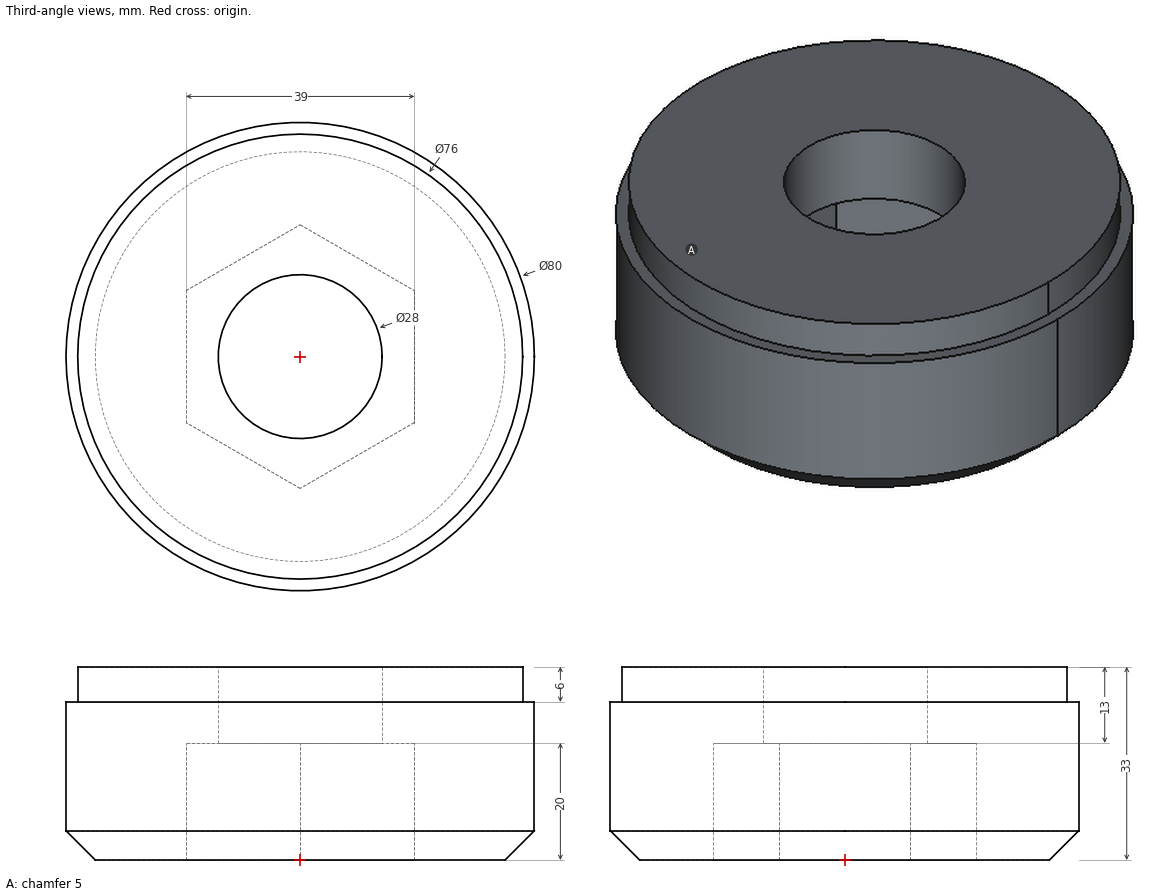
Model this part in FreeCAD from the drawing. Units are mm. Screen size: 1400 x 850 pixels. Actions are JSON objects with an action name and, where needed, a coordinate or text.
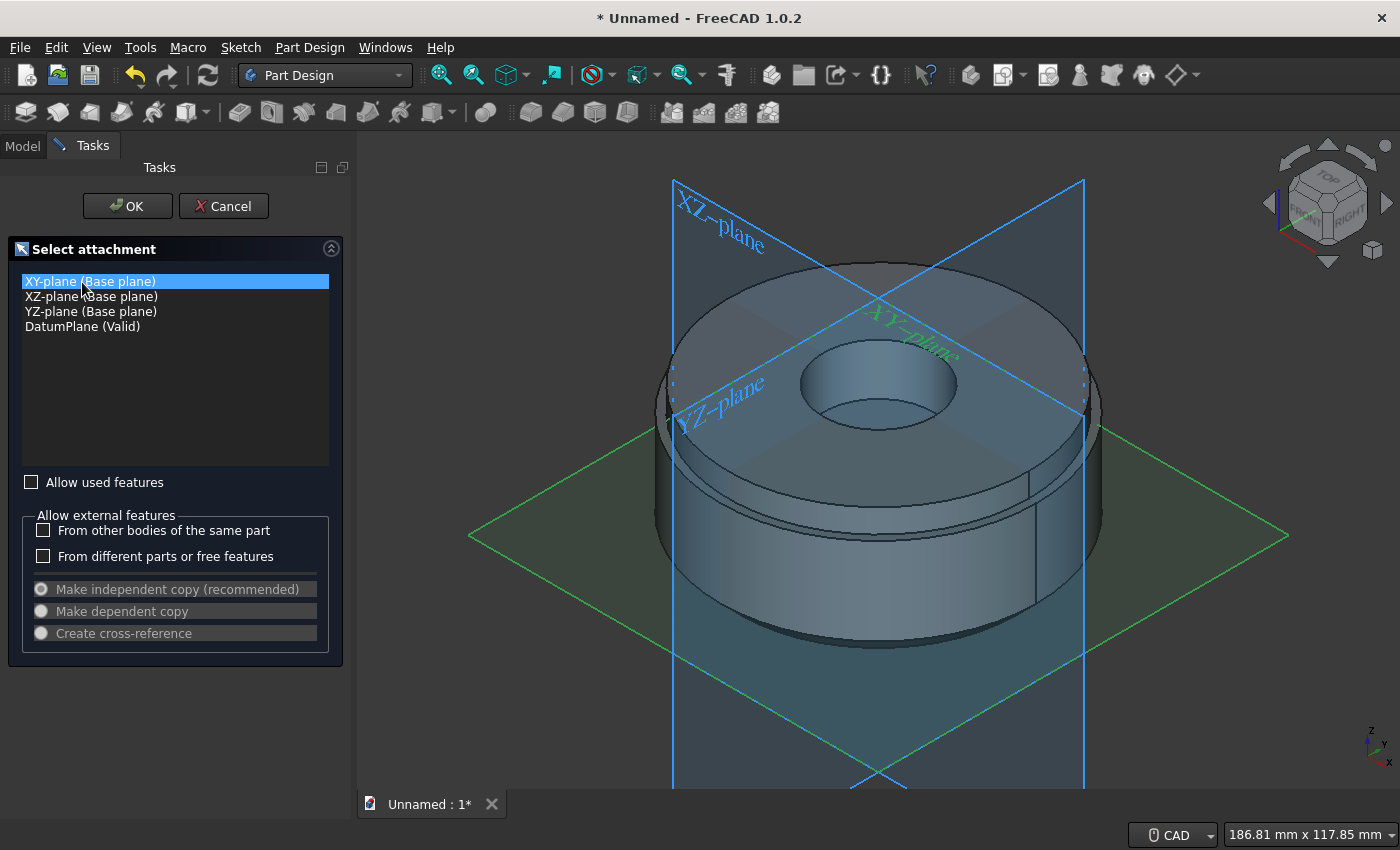
{"action": "left_click", "coordinate": [128, 206]}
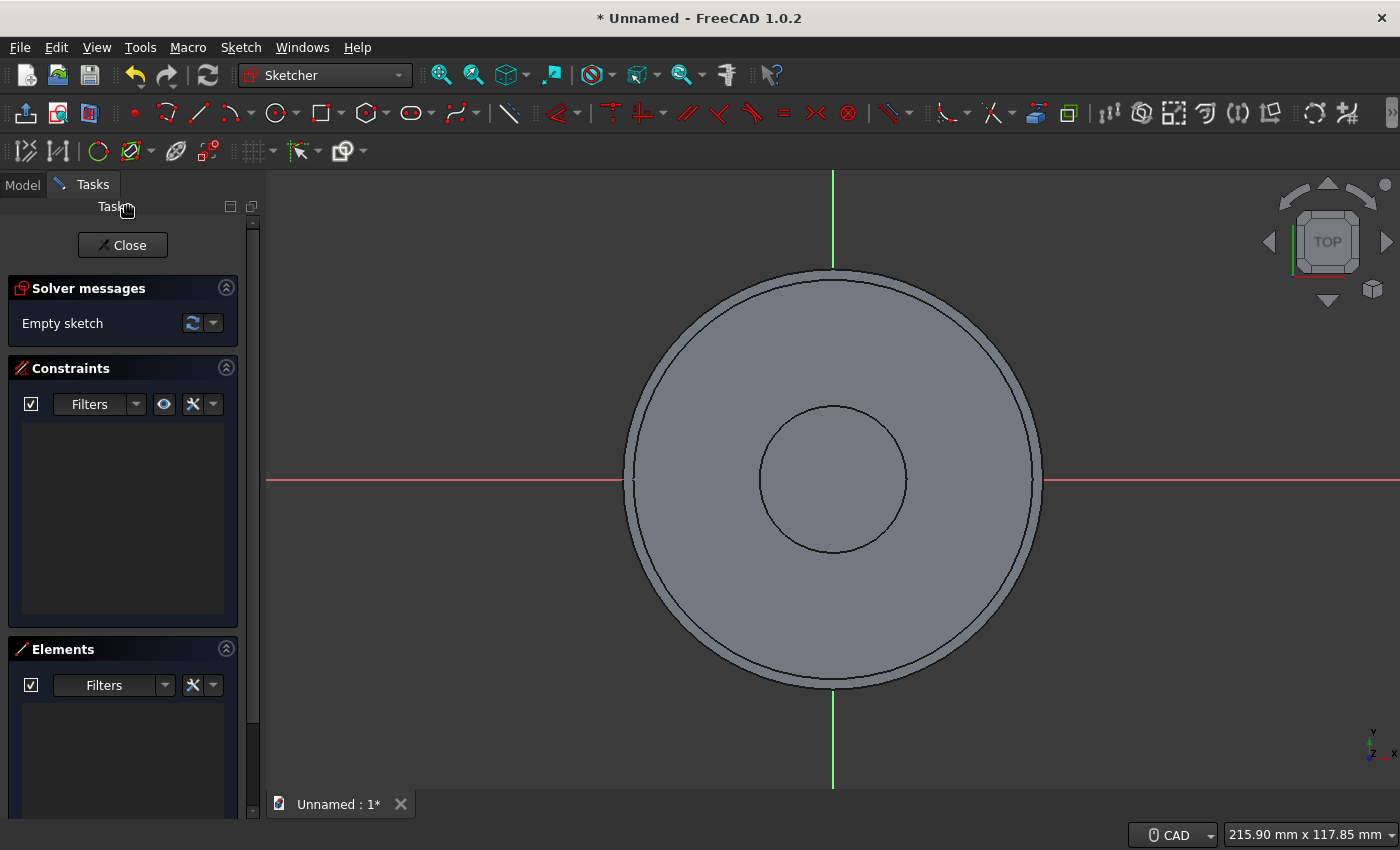
{"action": "left_click", "coordinate": [90, 114]}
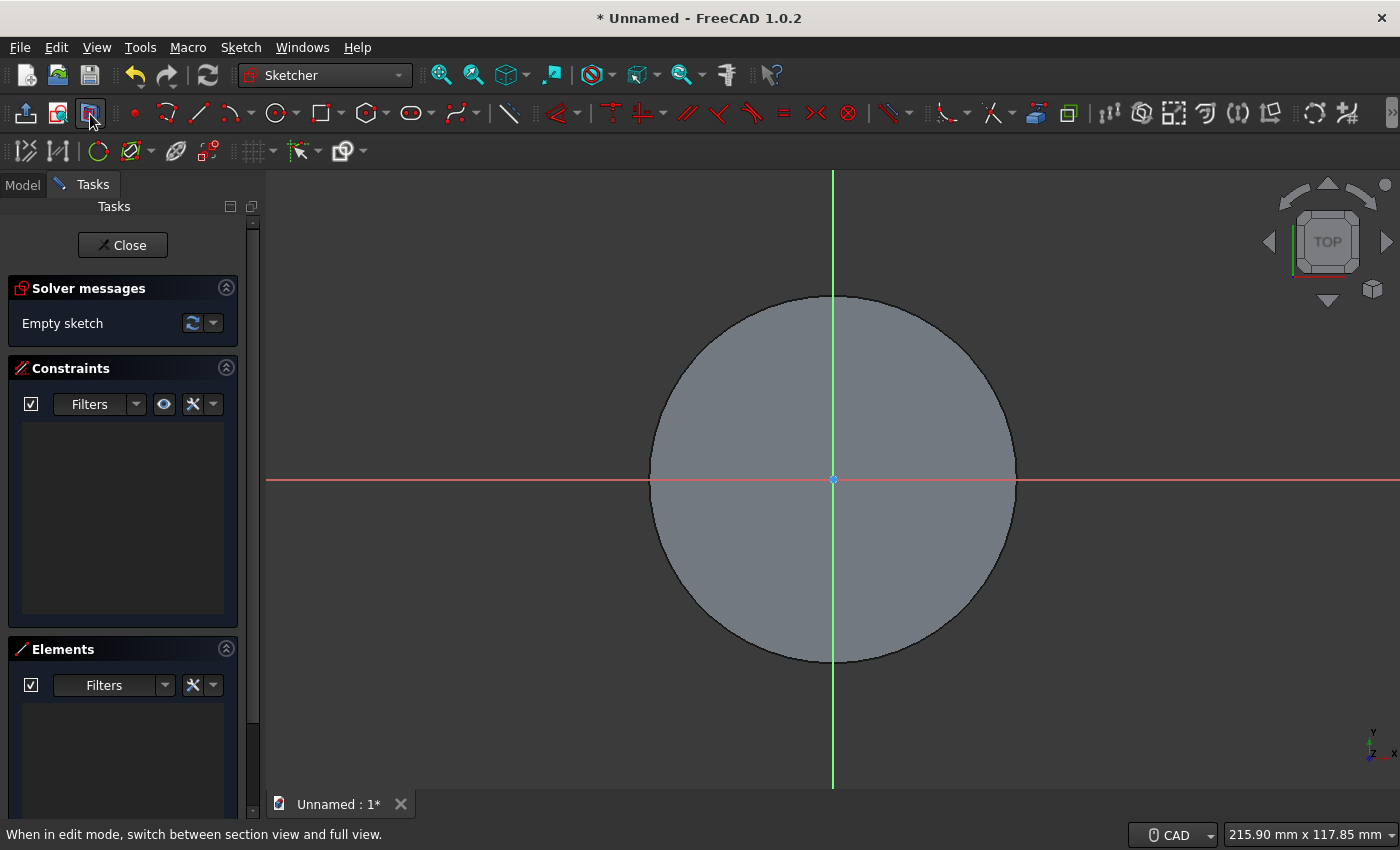
{"action": "scroll", "coordinate": [916, 480], "scroll_direction": "up", "scroll_amount": 3}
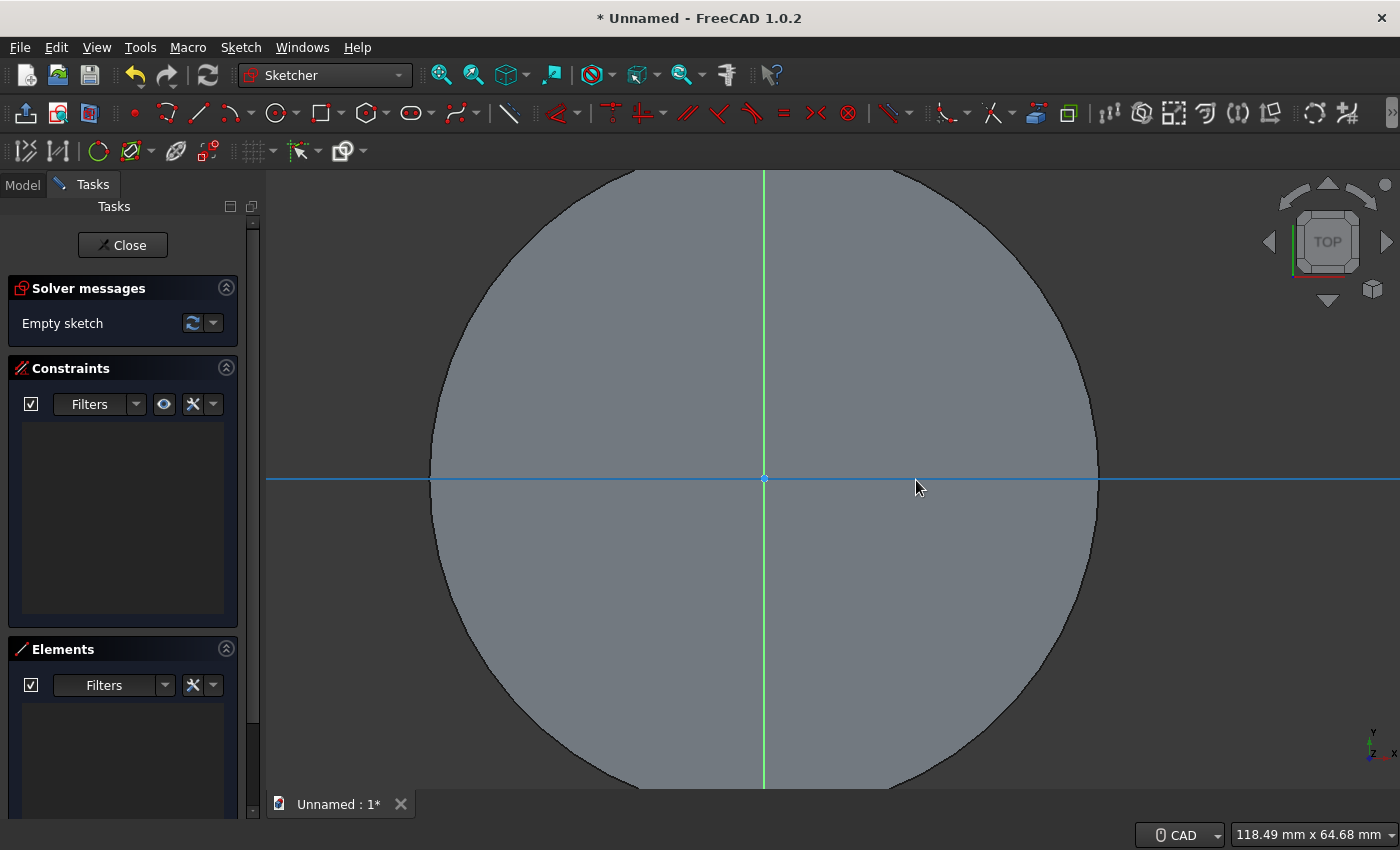
{"action": "left_click", "coordinate": [366, 114]}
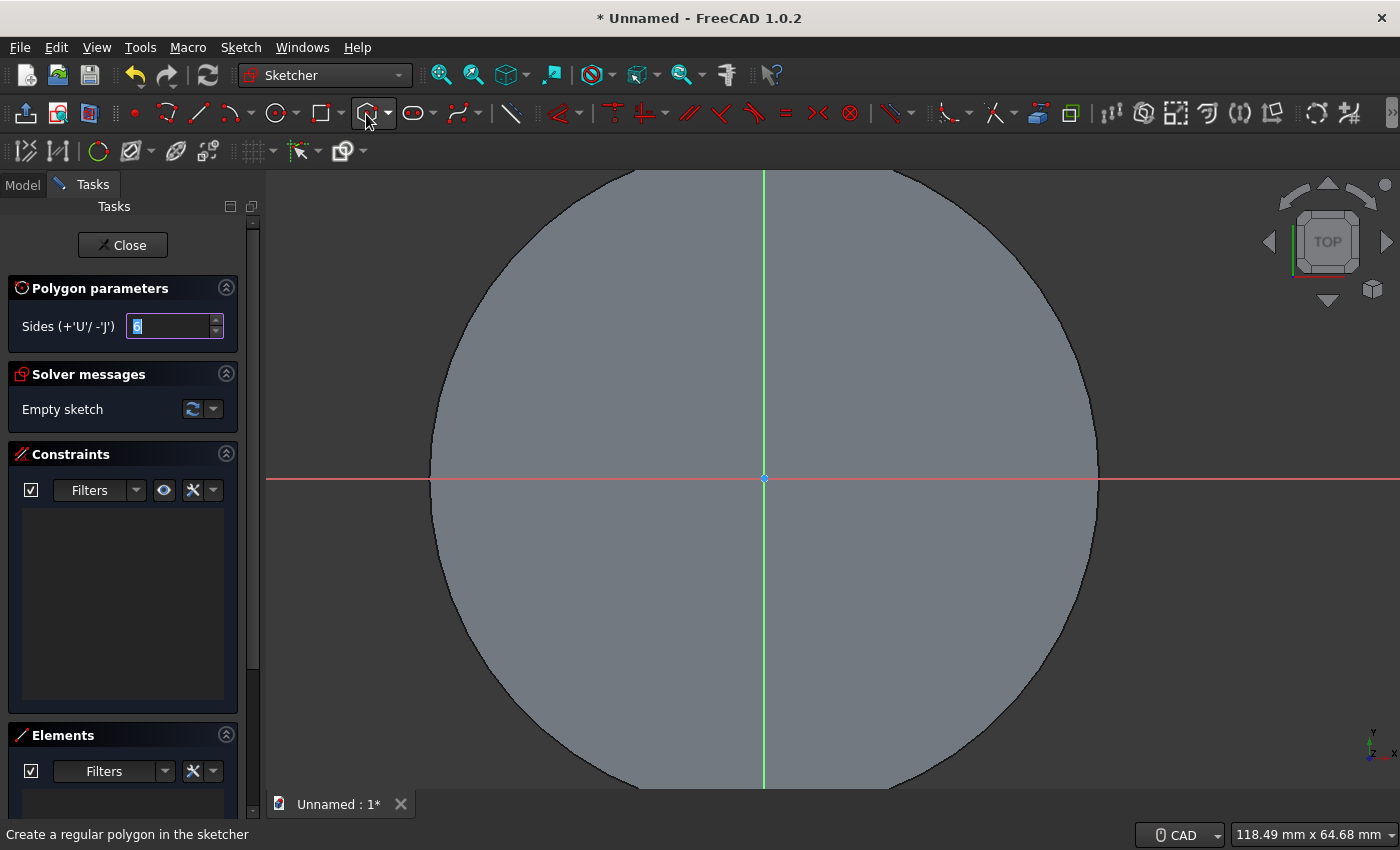
{"action": "left_click", "coordinate": [764, 479]}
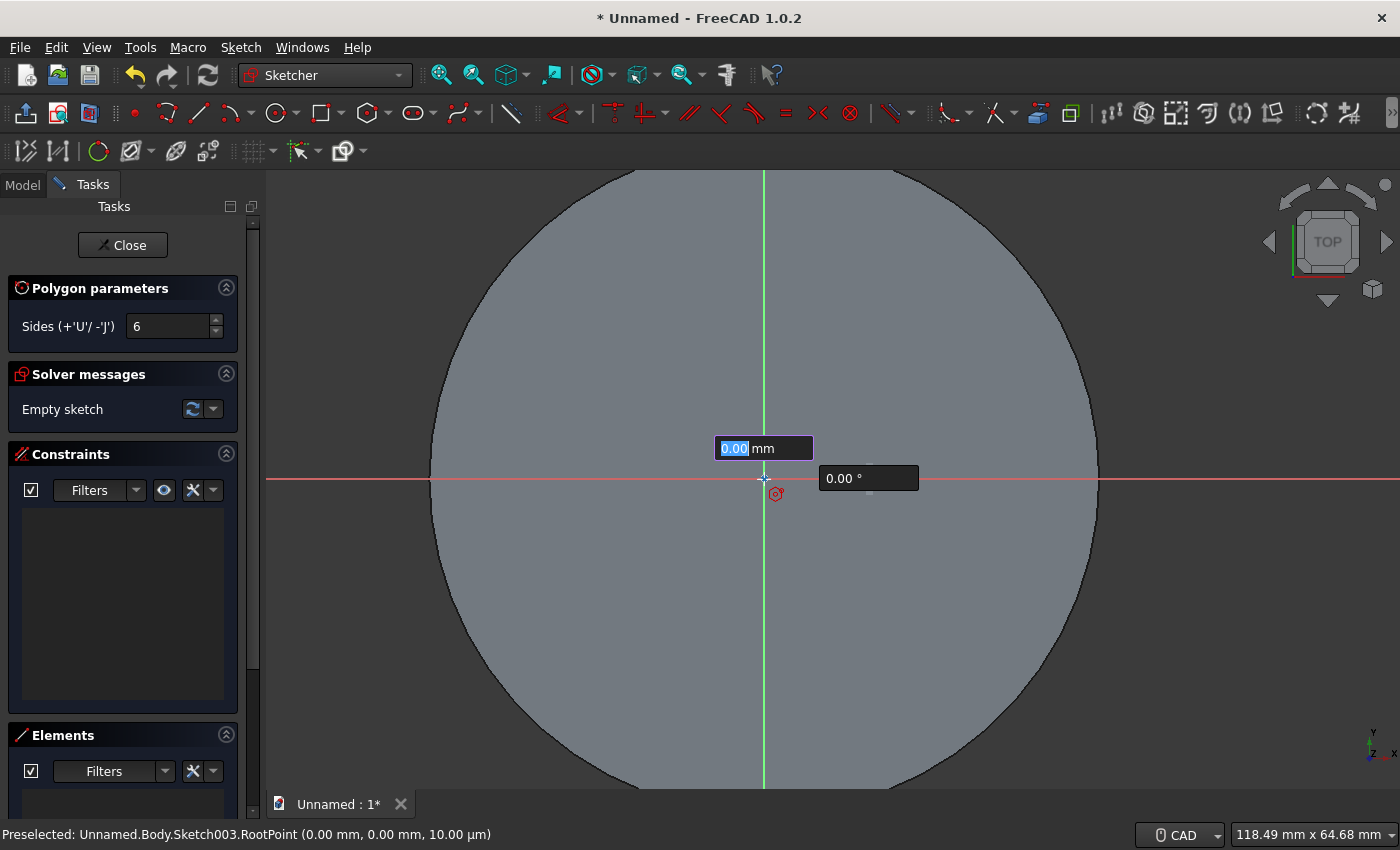
{"action": "left_click", "coordinate": [764, 694]}
{"action": "right_click", "coordinate": [764, 694]}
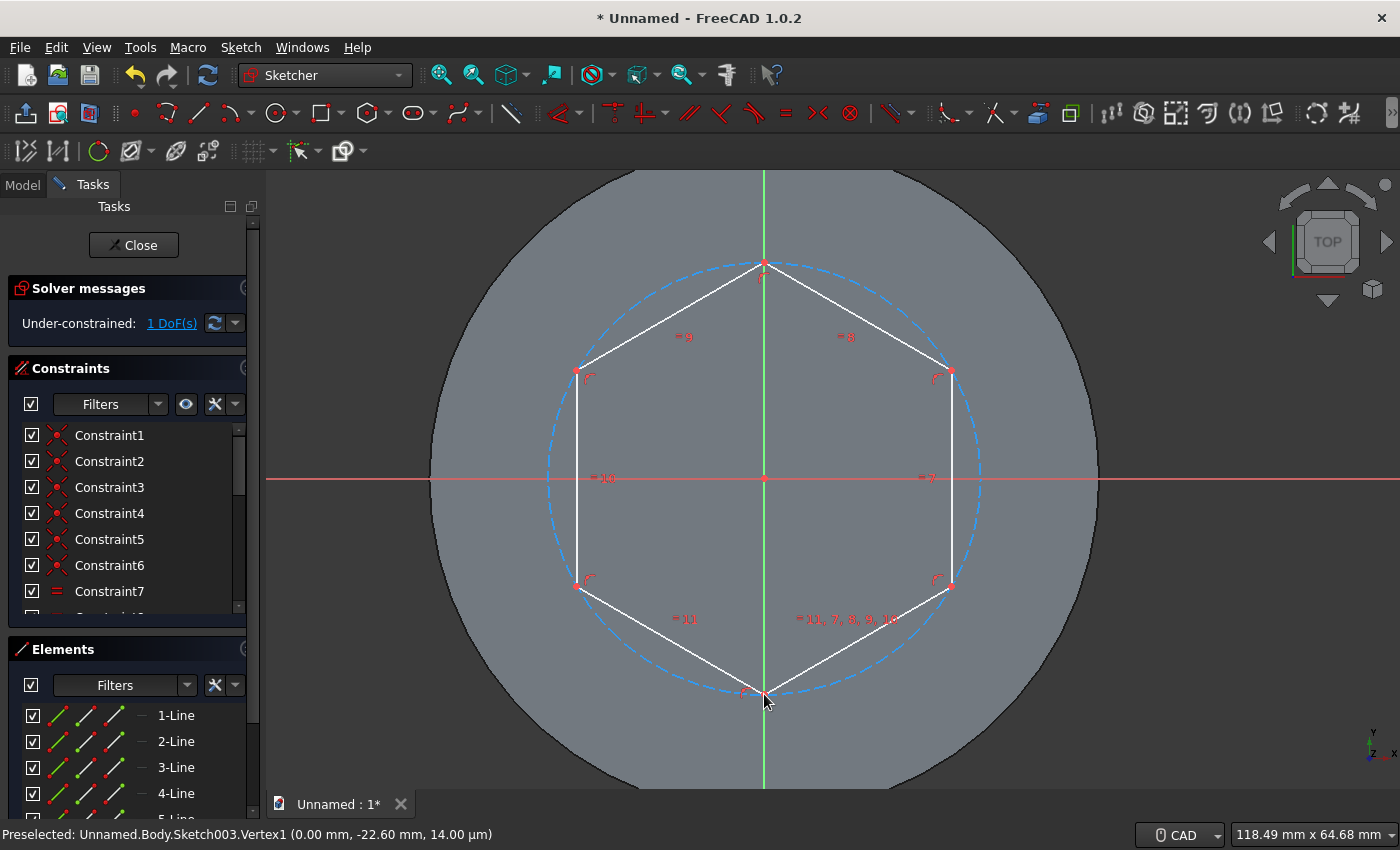
{"action": "left_click", "coordinate": [558, 114]}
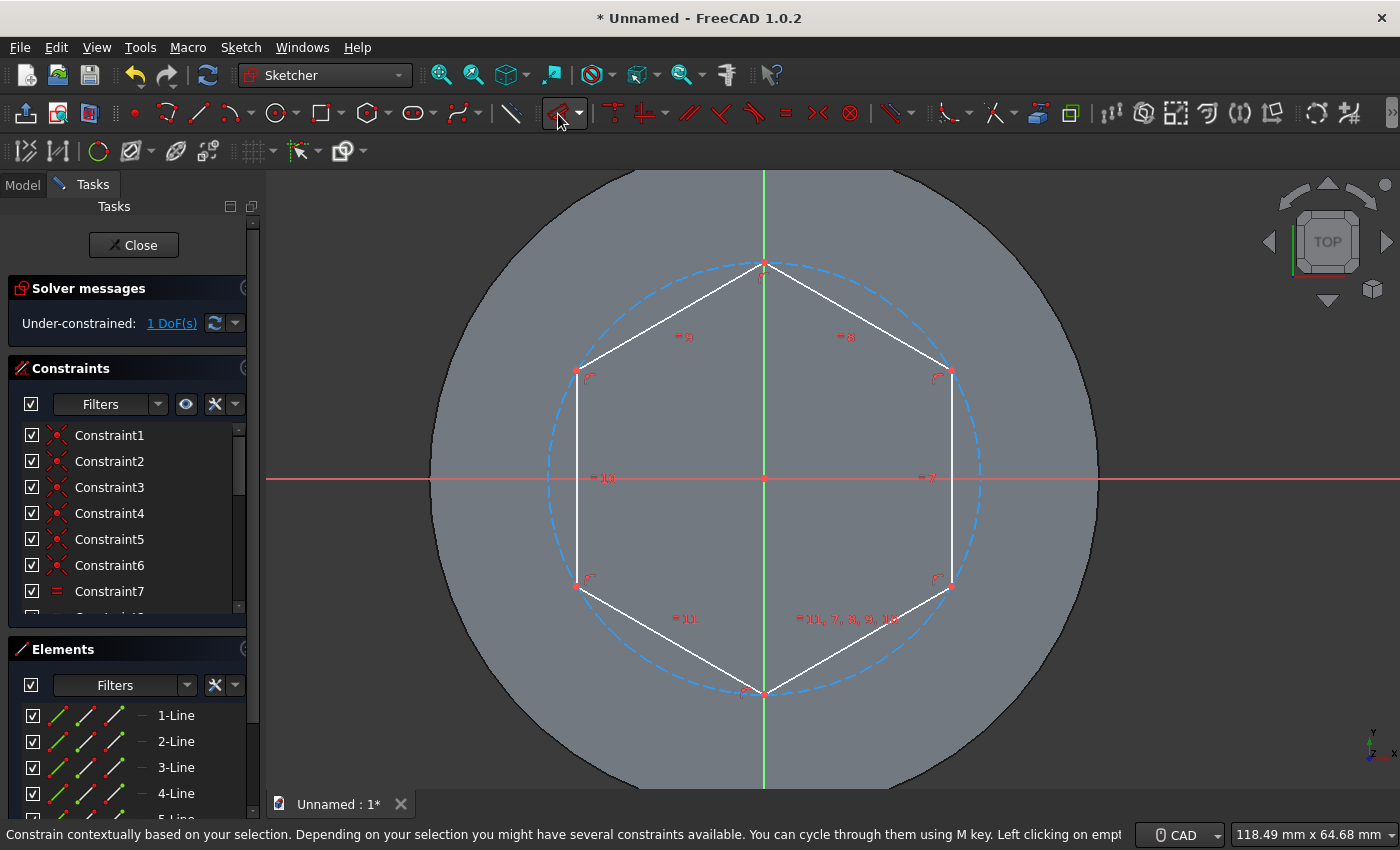
{"action": "left_click", "coordinate": [577, 371]}